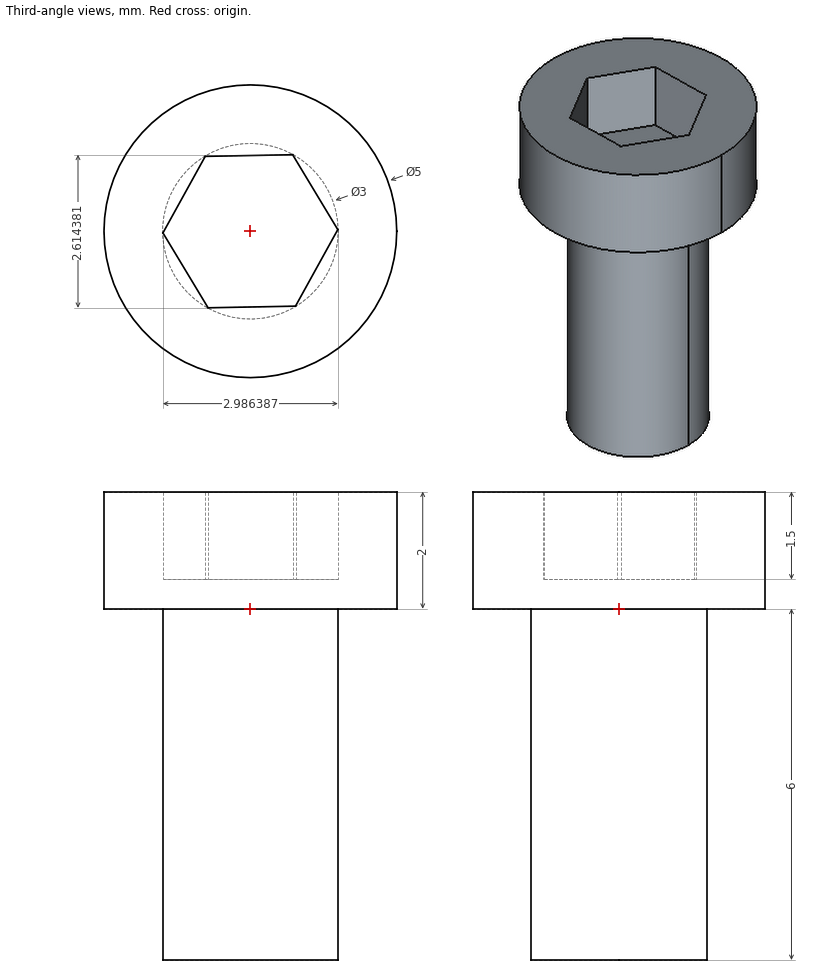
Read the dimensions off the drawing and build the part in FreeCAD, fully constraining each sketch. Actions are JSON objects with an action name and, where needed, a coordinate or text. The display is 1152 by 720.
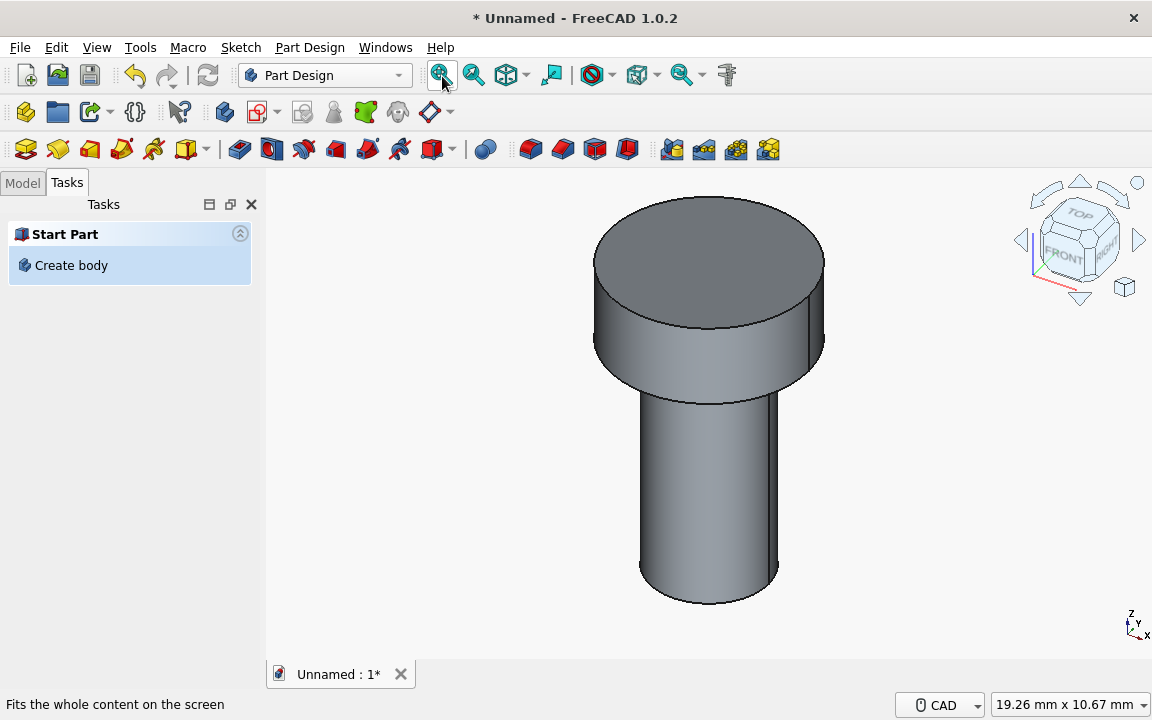
{"action": "left_click", "coordinate": [709, 262]}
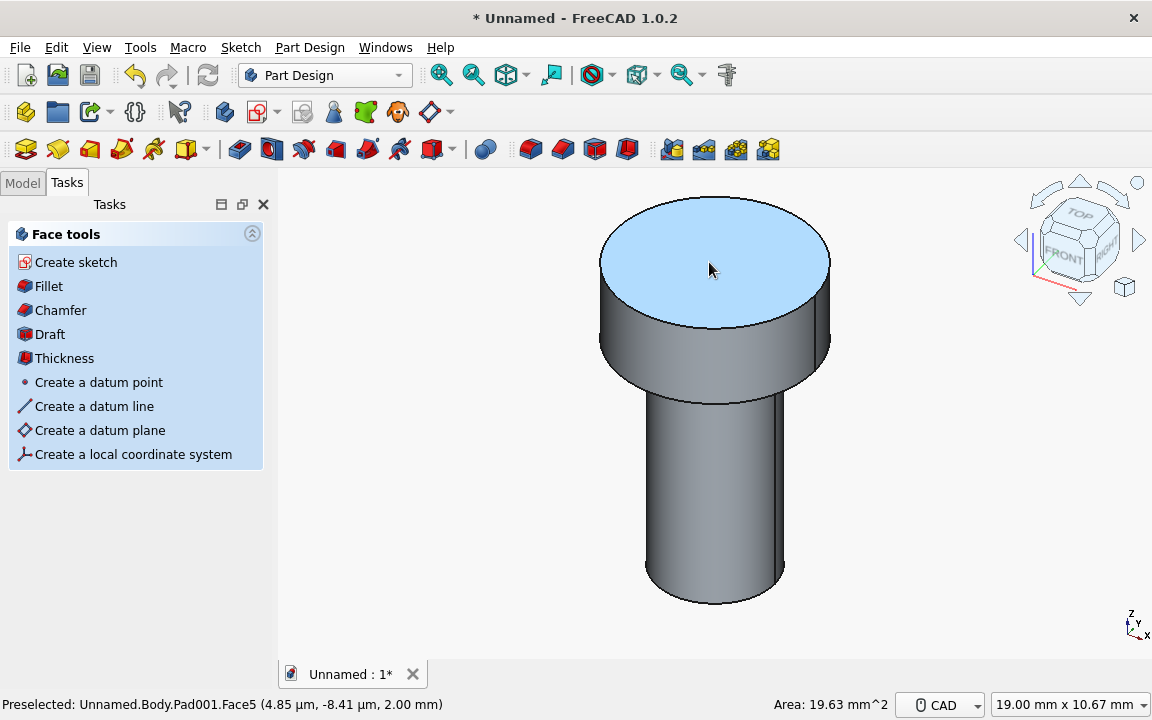
{"action": "left_click", "coordinate": [258, 112]}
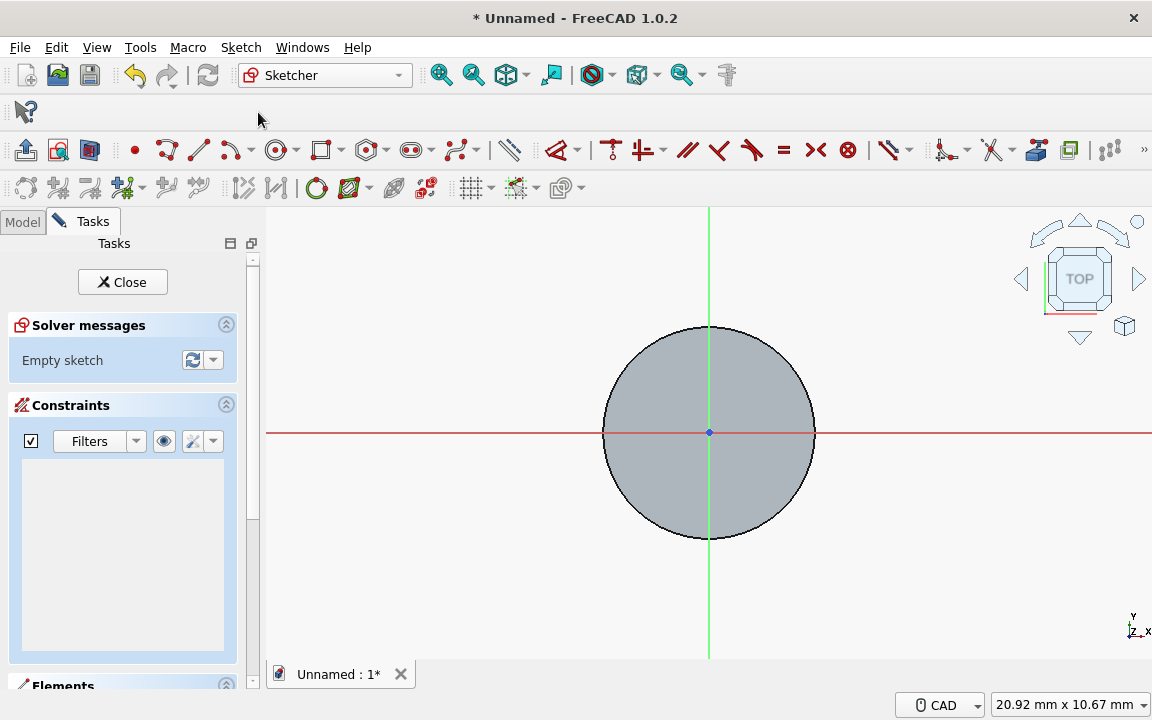
{"action": "scroll", "coordinate": [749, 433], "scroll_direction": "up", "scroll_amount": 5}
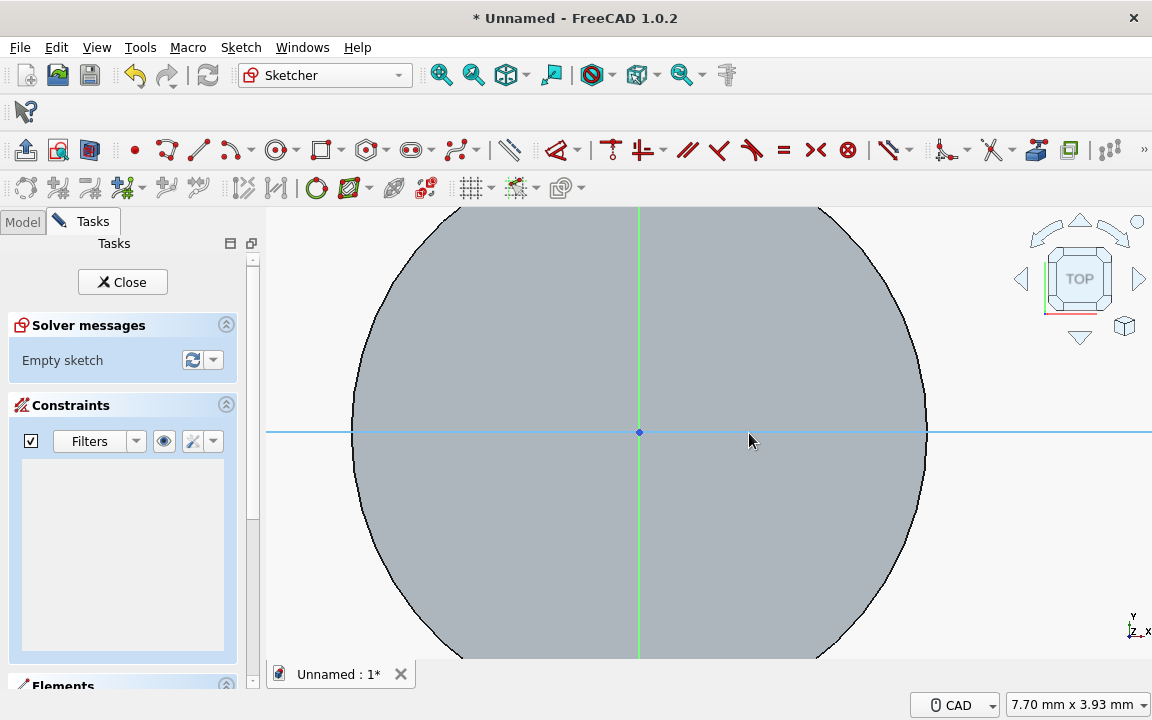
{"action": "key", "text": "g p 6"}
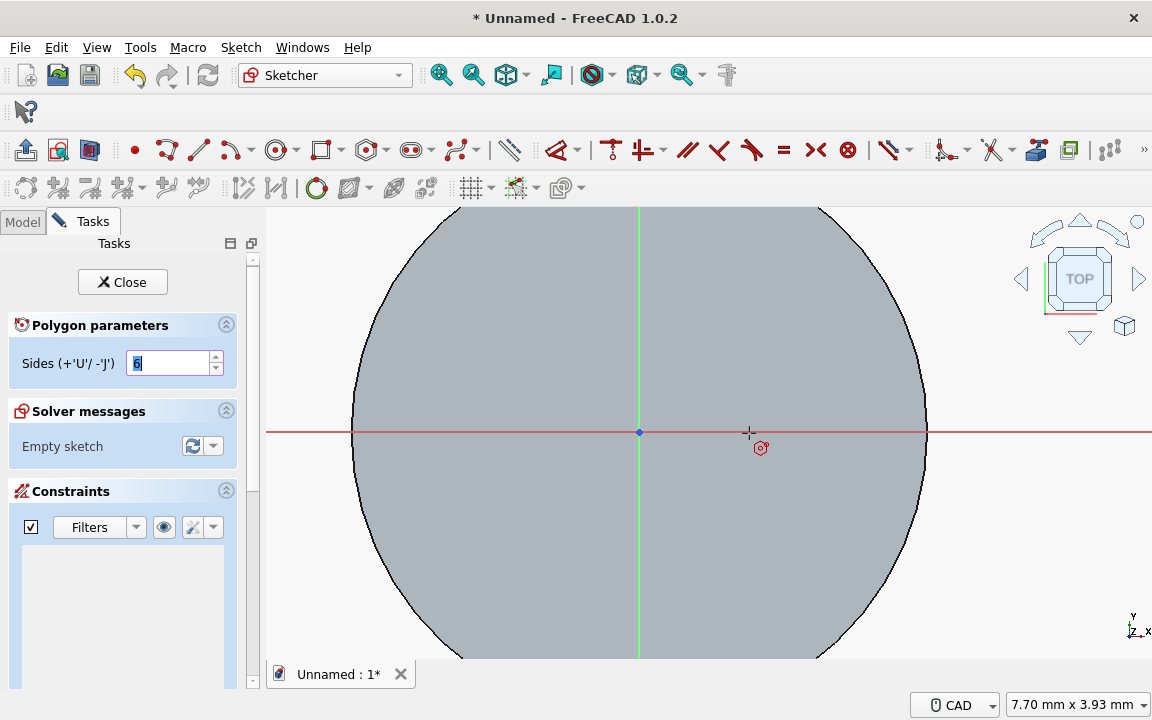
{"action": "left_click", "coordinate": [639, 432]}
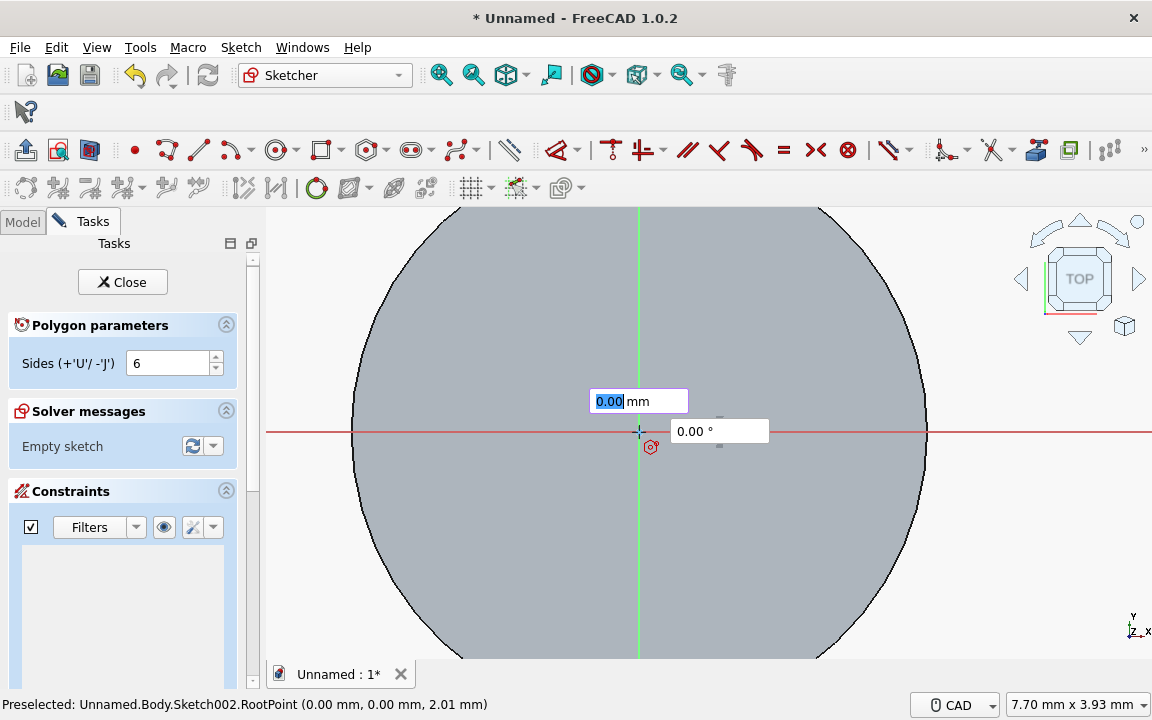
{"action": "left_click", "coordinate": [551, 285]}
{"action": "right_click", "coordinate": [551, 285]}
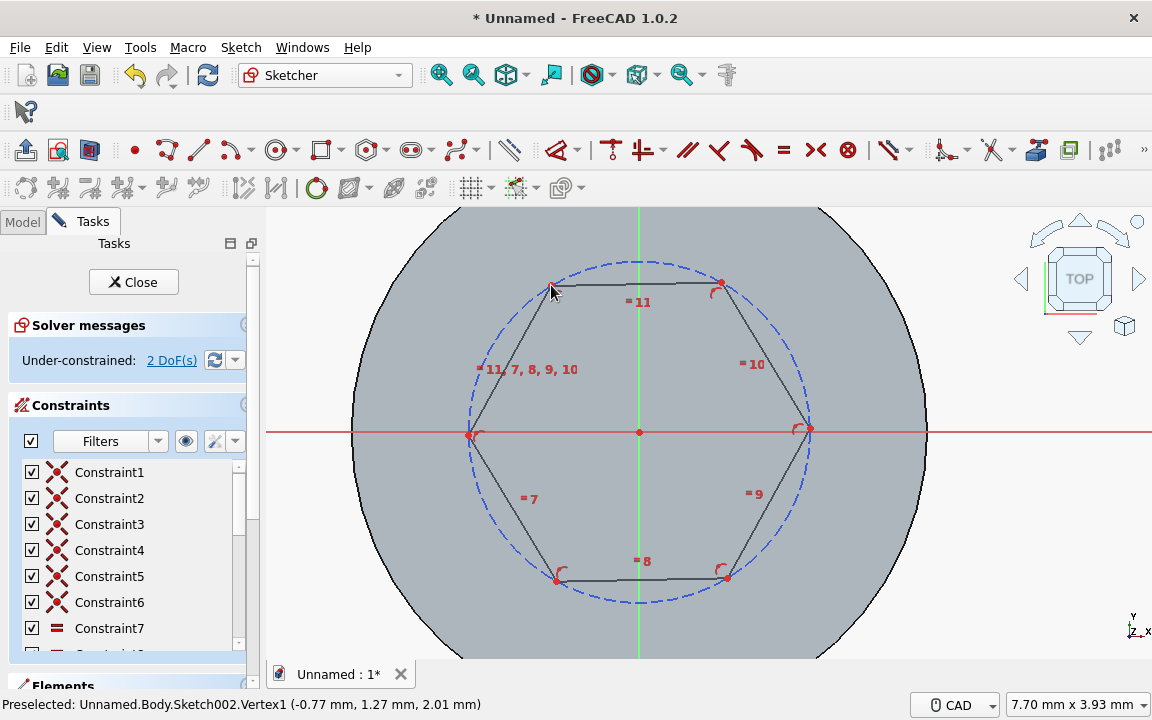
{"action": "key", "text": "d"}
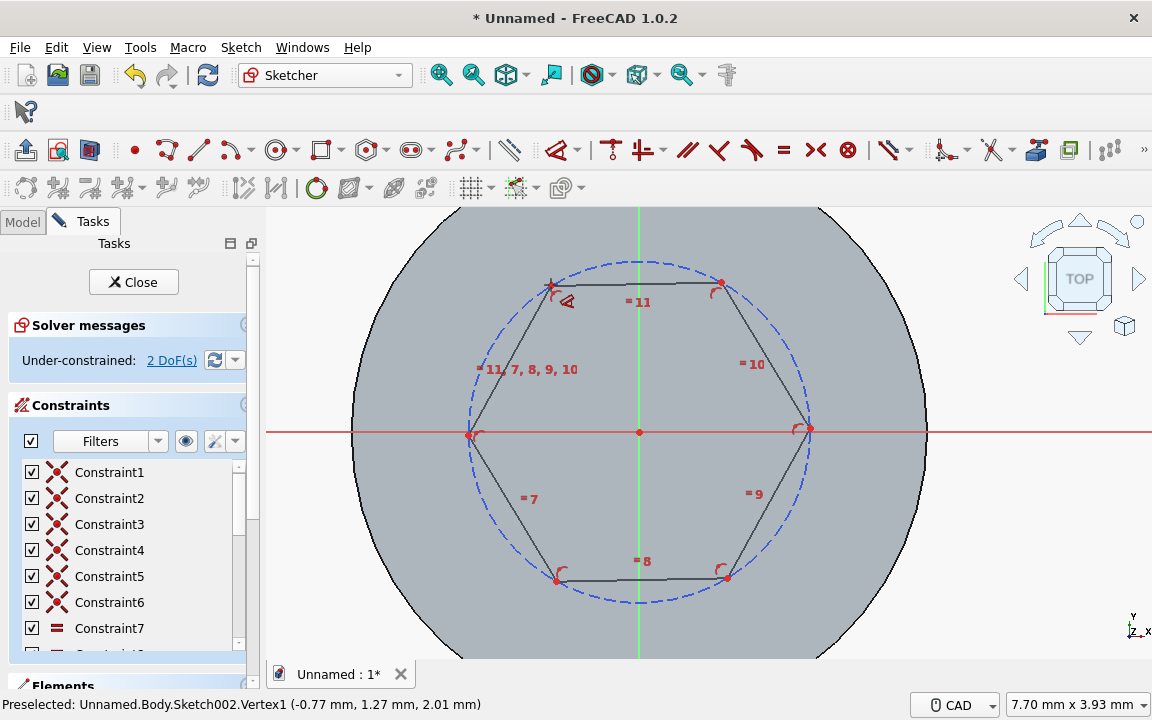
{"action": "left_click", "coordinate": [469, 436]}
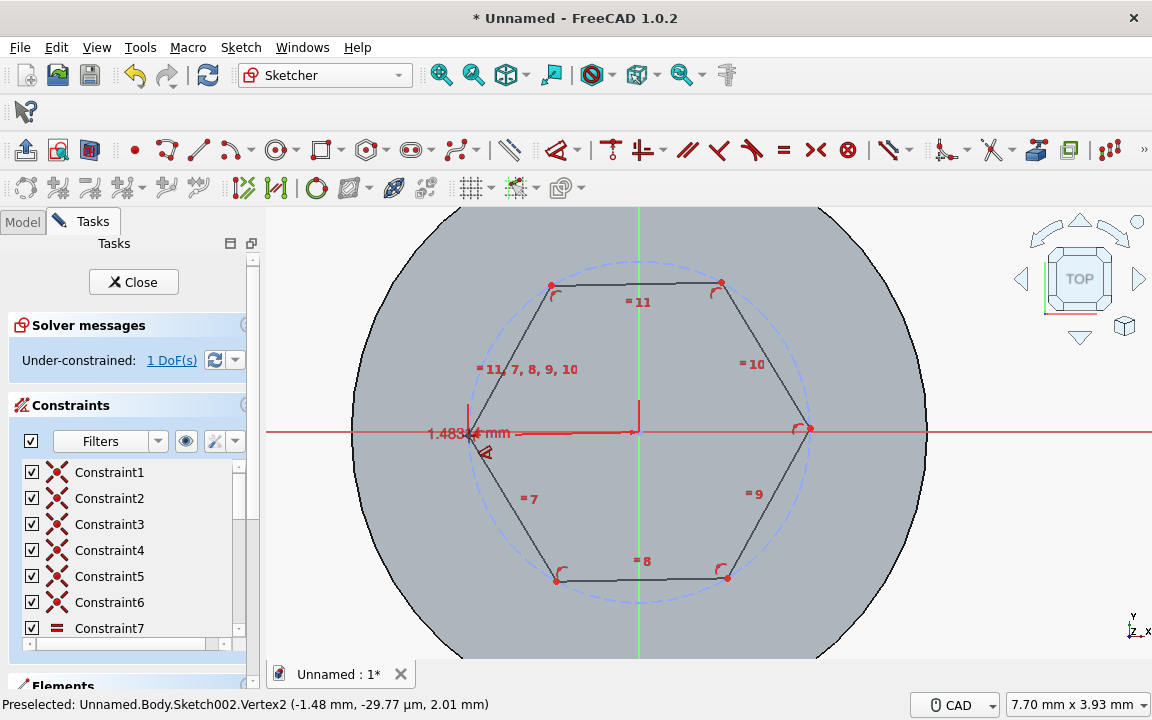
{"action": "left_click", "coordinate": [810, 429]}
{"action": "left_click", "coordinate": [561, 470]}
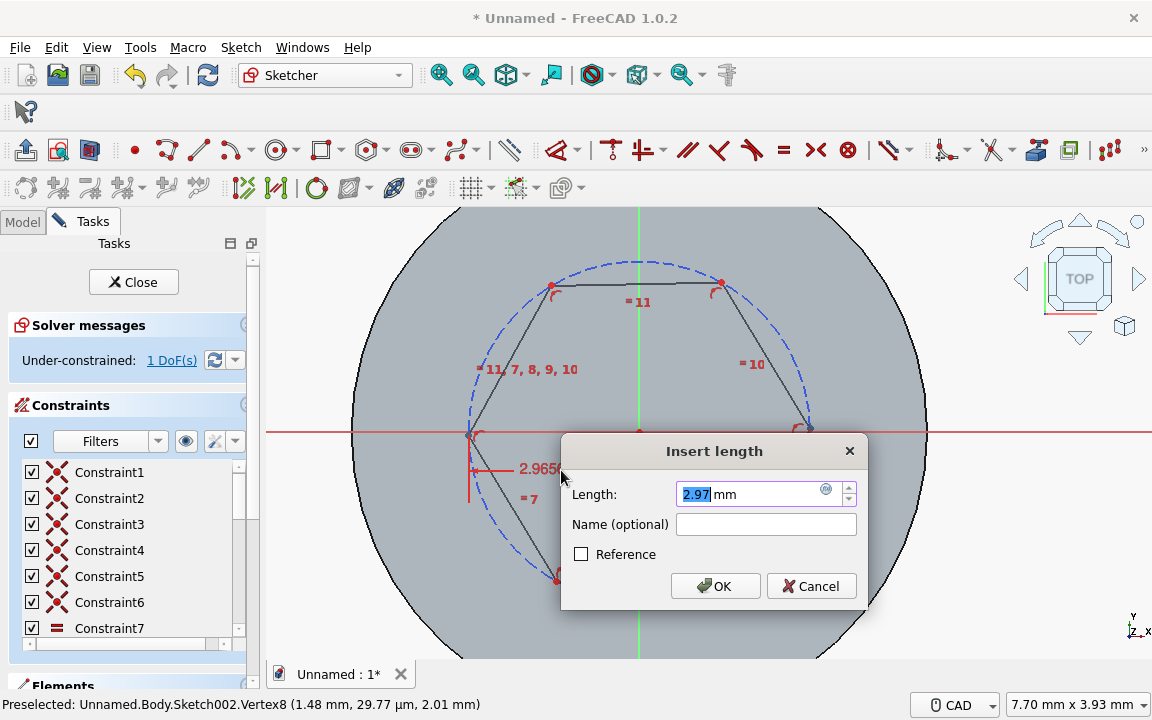
{"action": "type", "text": "2.986387"}
{"action": "key", "text": "Return"}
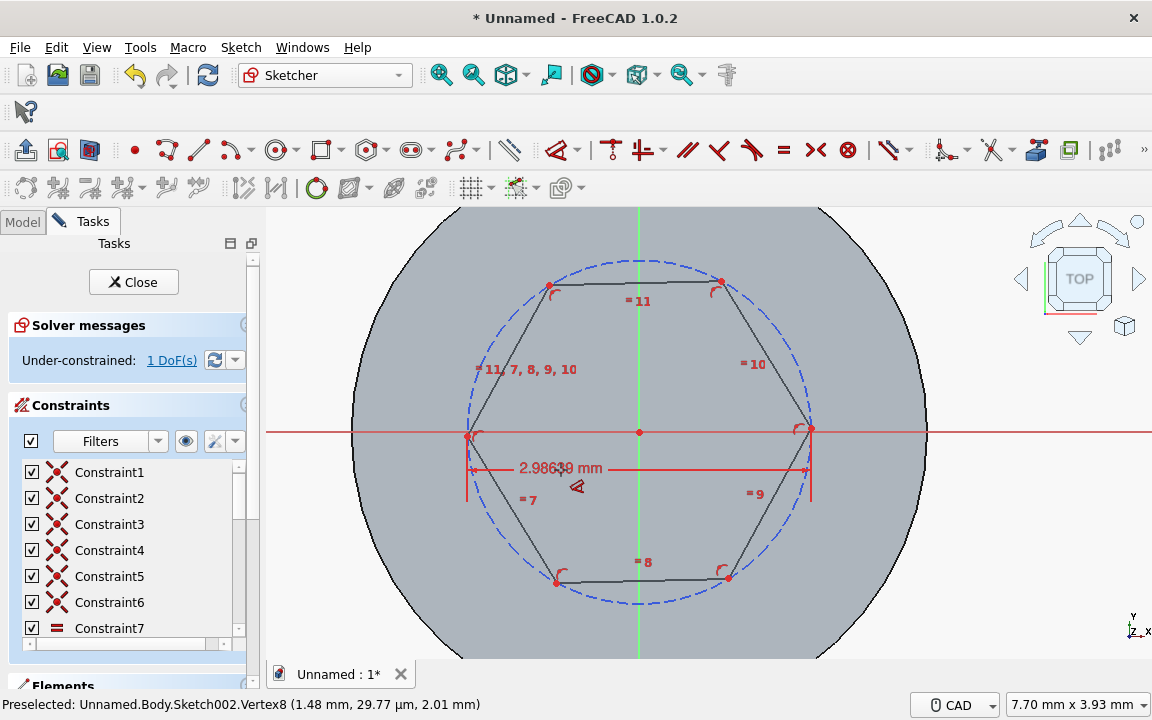
{"action": "left_click", "coordinate": [557, 583]}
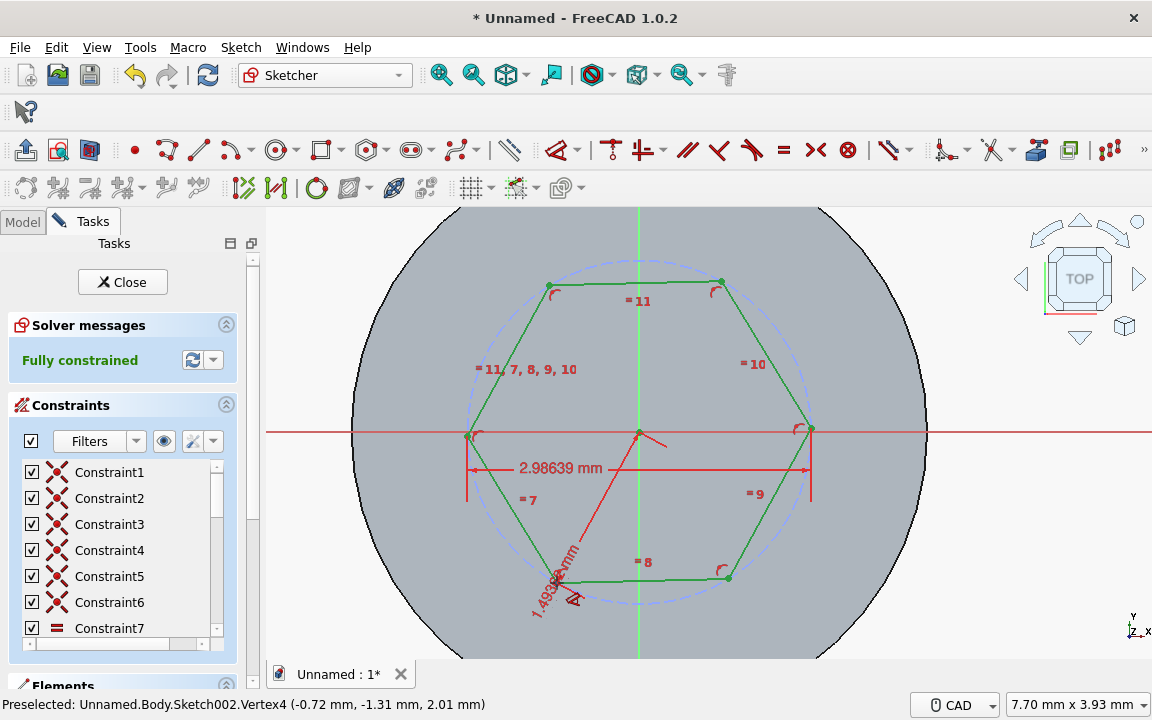
{"action": "left_click", "coordinate": [722, 281]}
{"action": "left_click", "coordinate": [756, 363]}